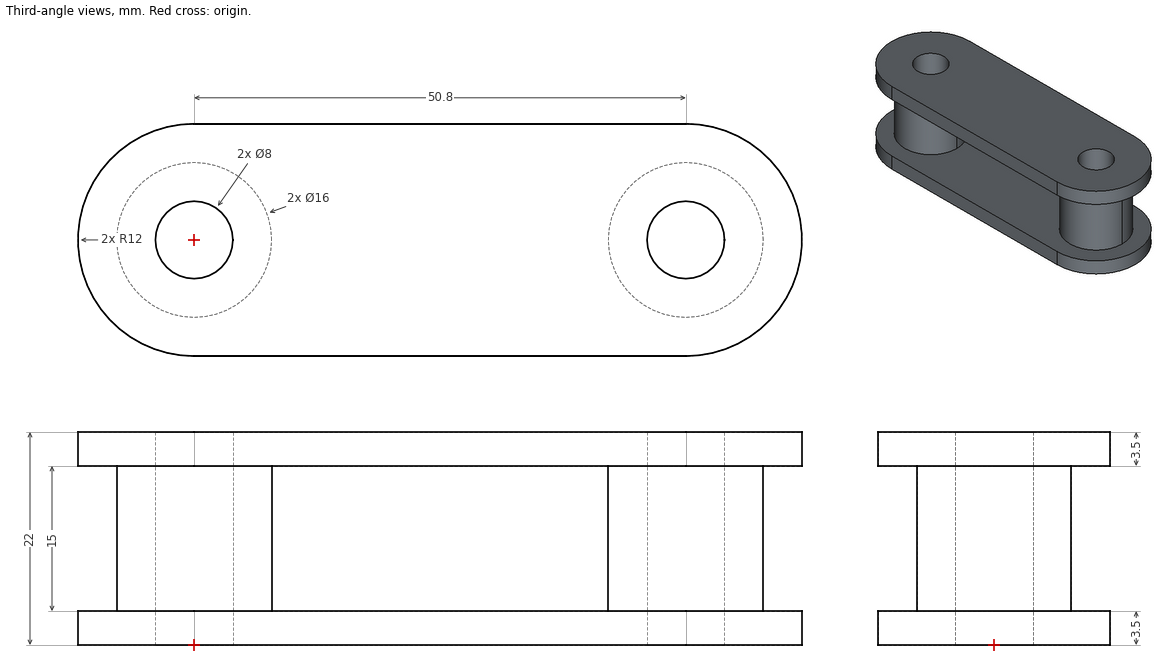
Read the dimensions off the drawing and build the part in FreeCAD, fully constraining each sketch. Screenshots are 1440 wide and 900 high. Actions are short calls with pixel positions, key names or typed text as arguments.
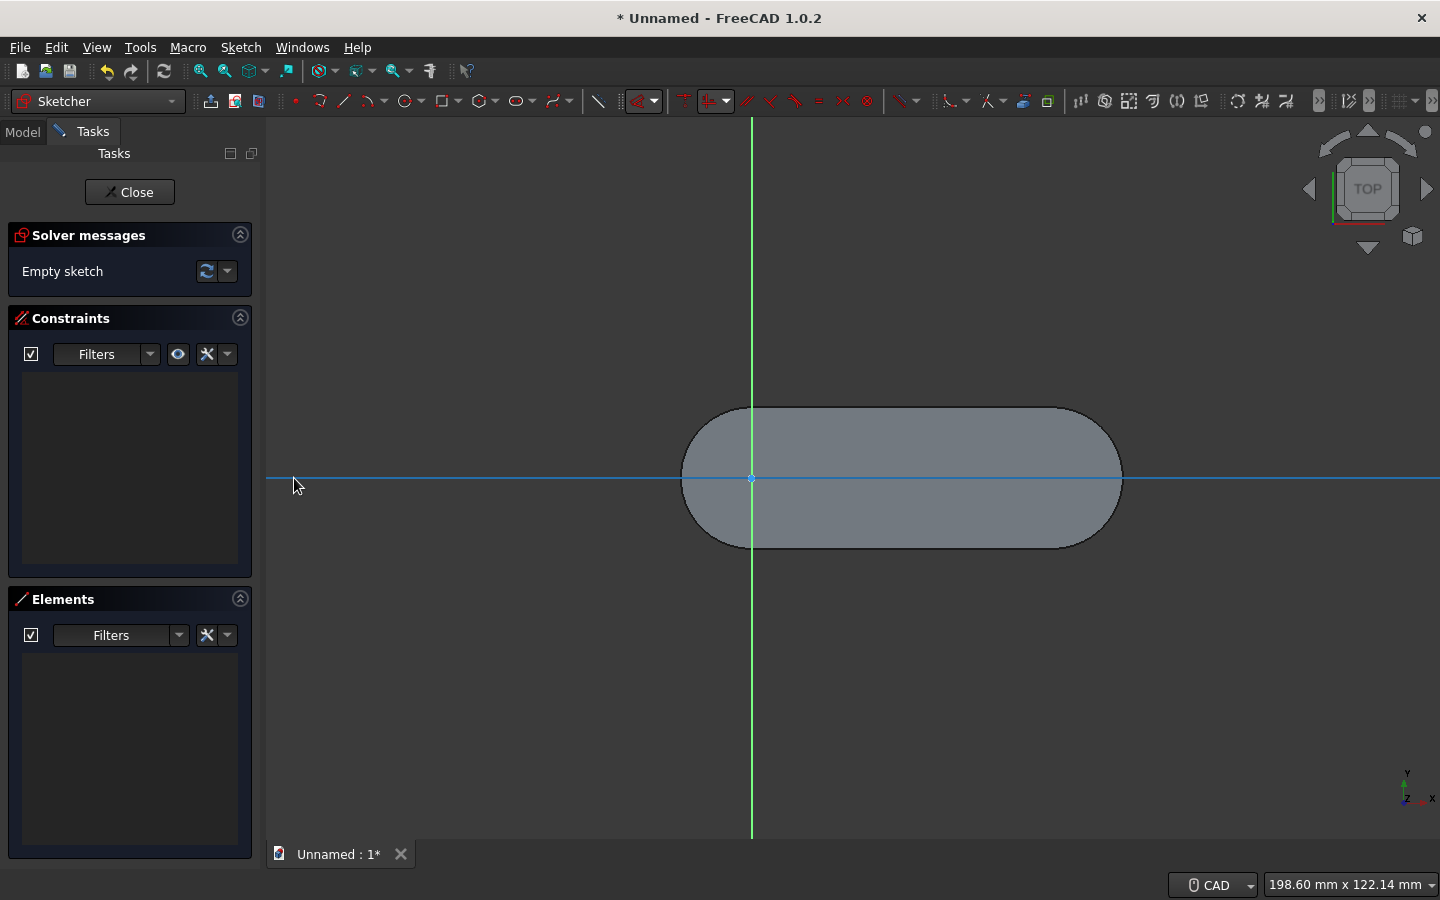
scroll(1045, 478, up, 3)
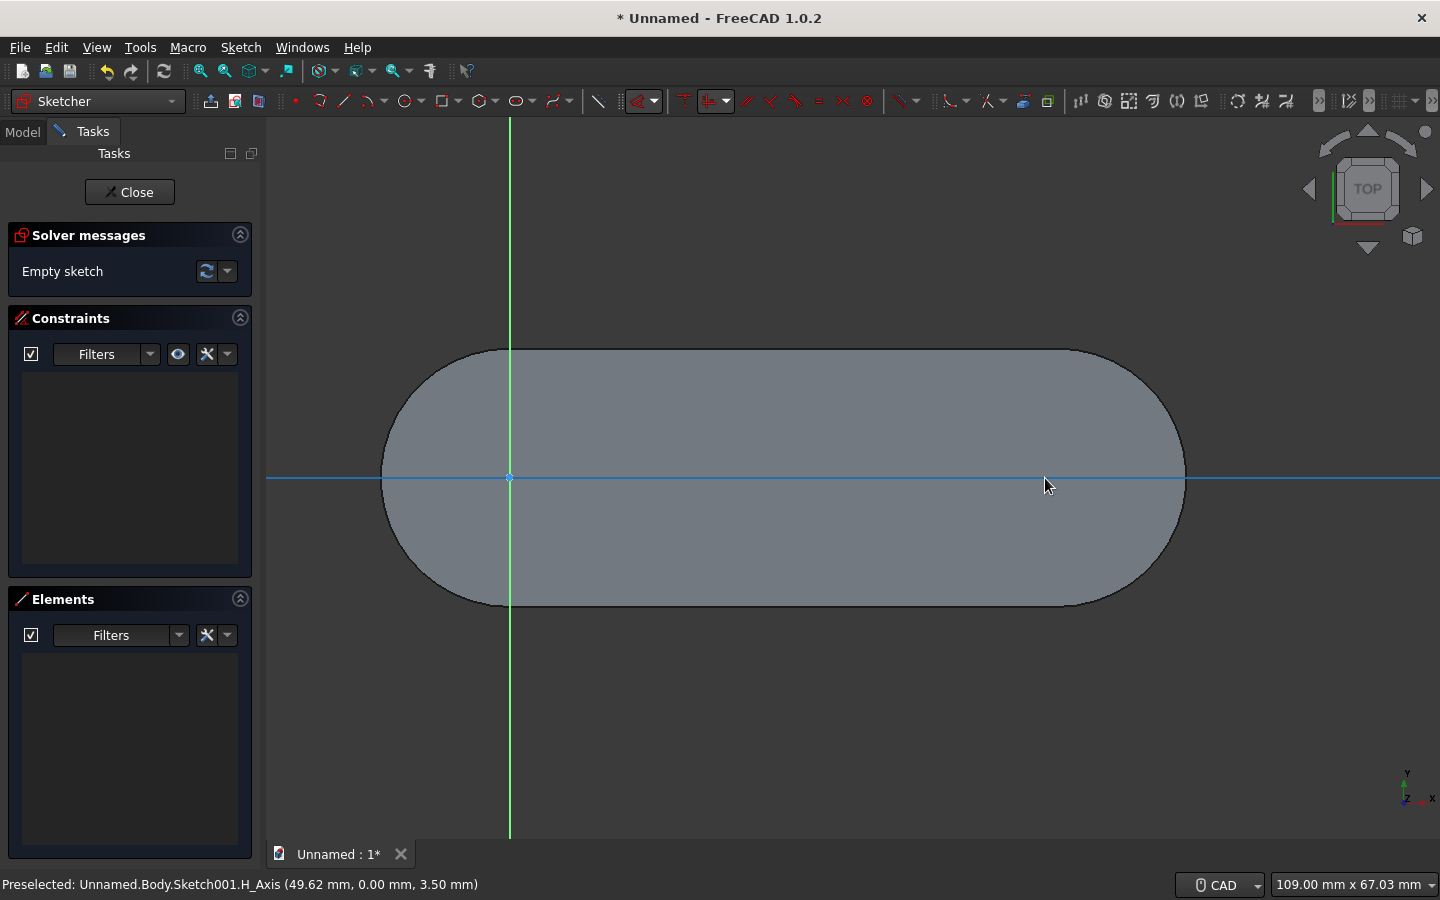
click(406, 102)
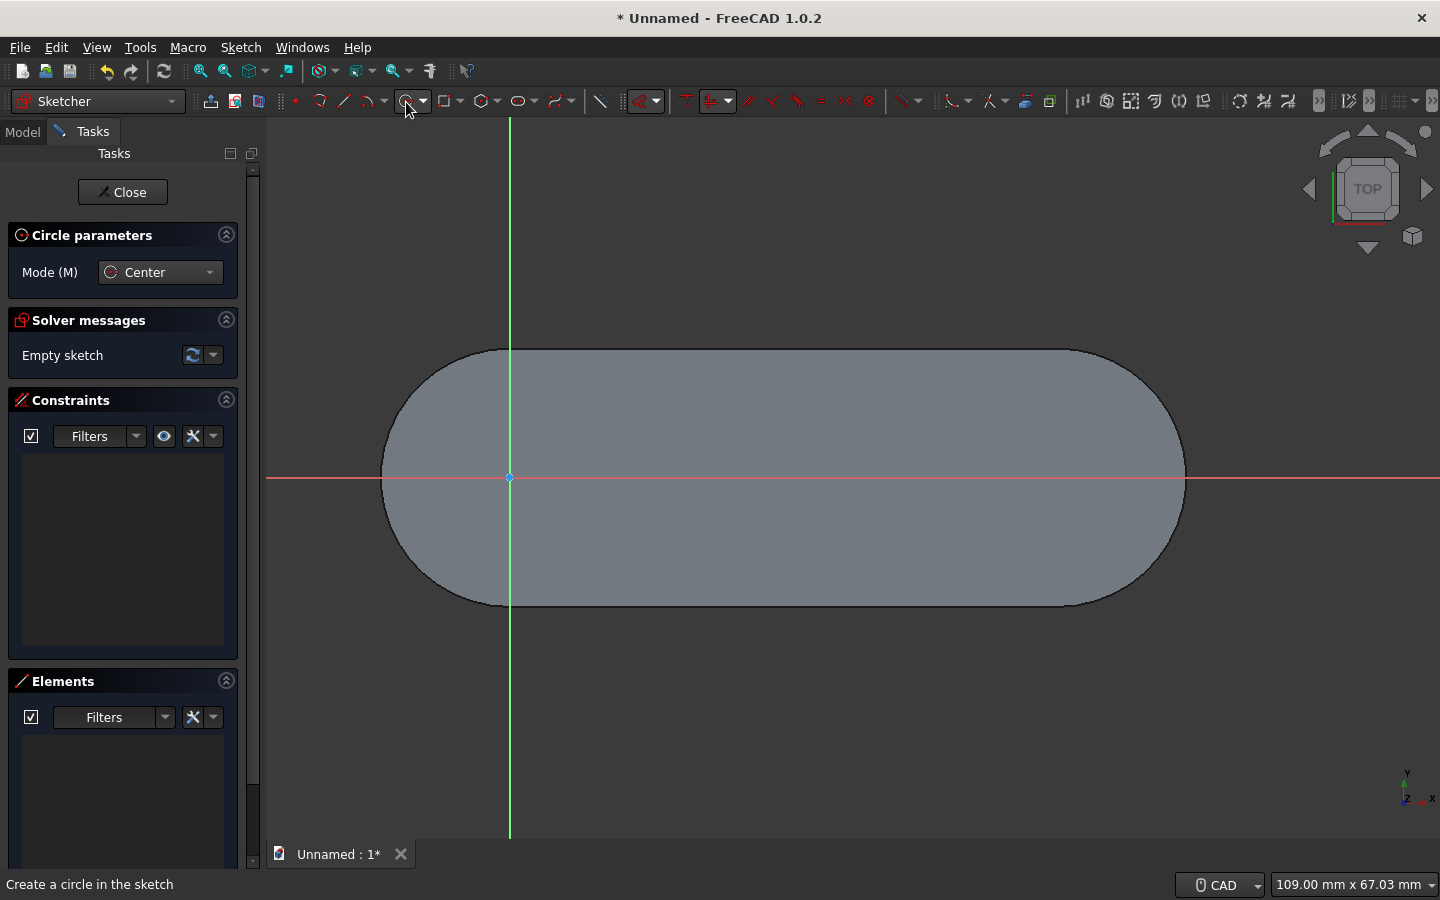
click(510, 478)
move(571, 417)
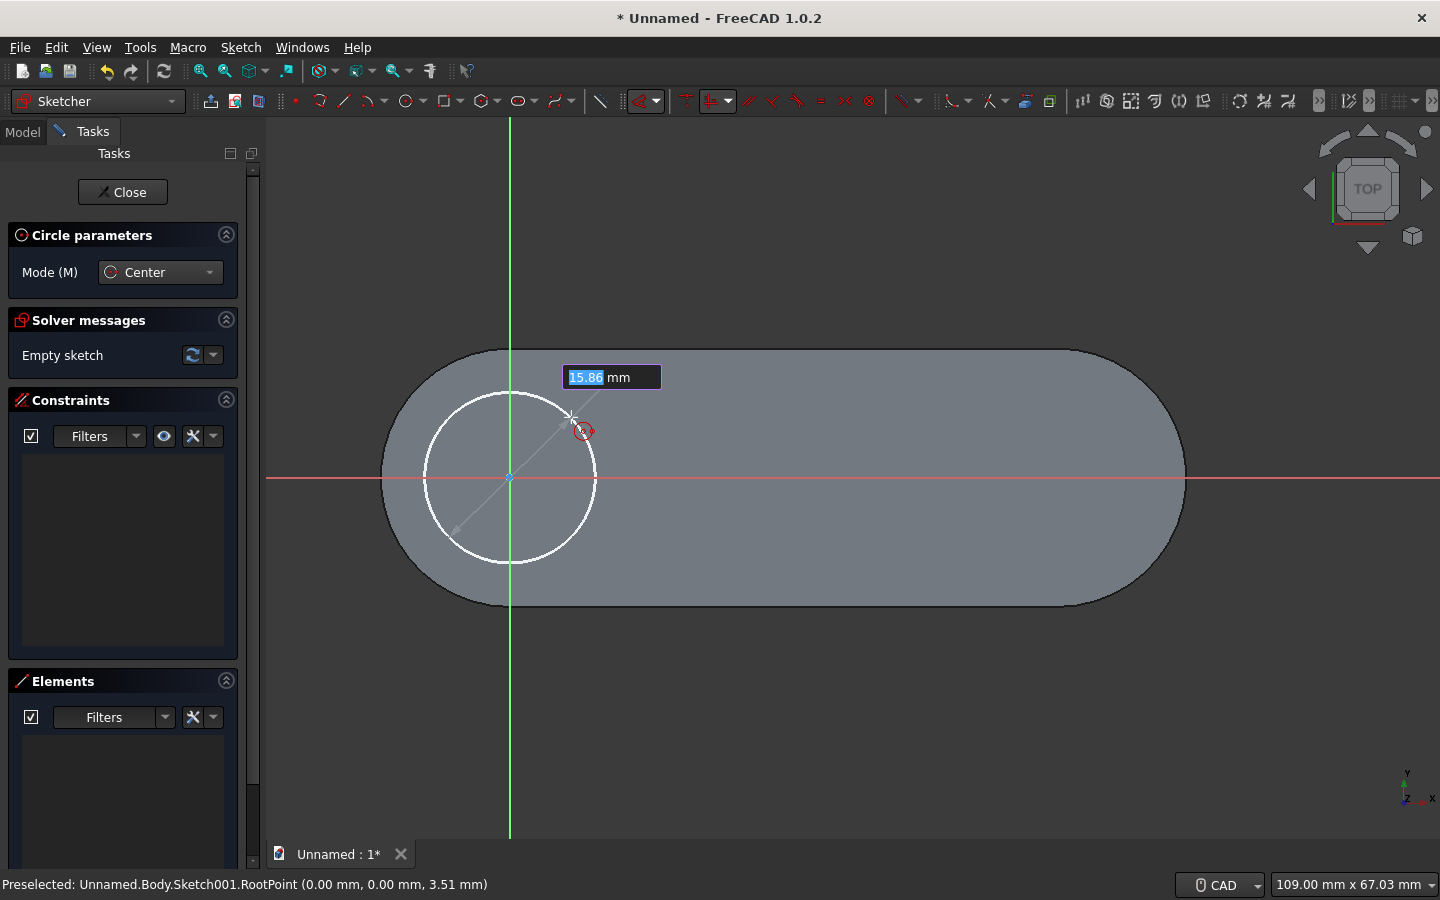
text(16)
key(Return)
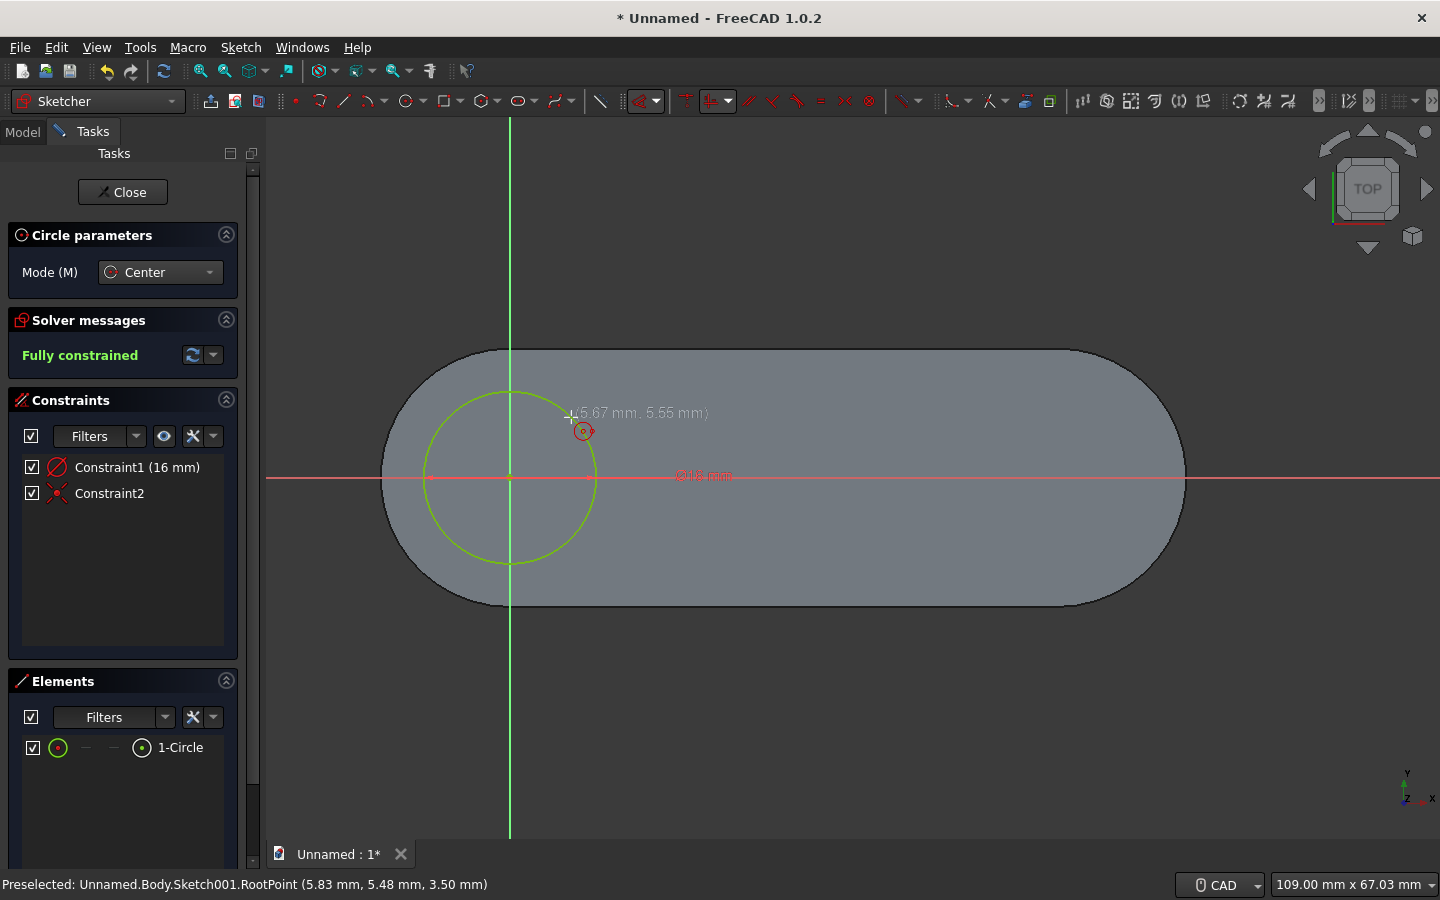
click(1057, 478)
move(1118, 417)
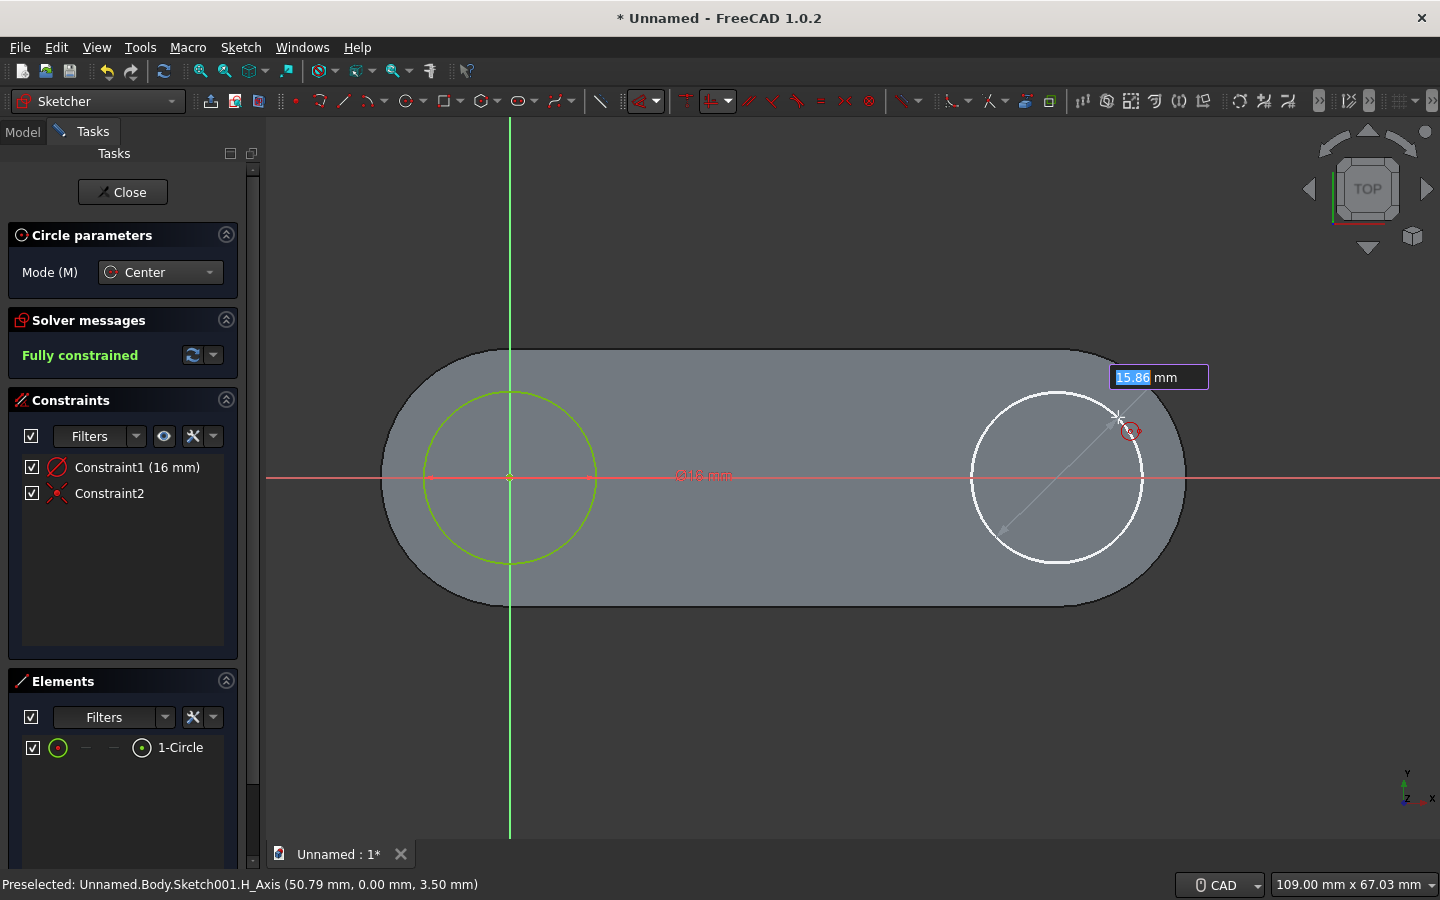
text(16)
key(Return)
key(Escape)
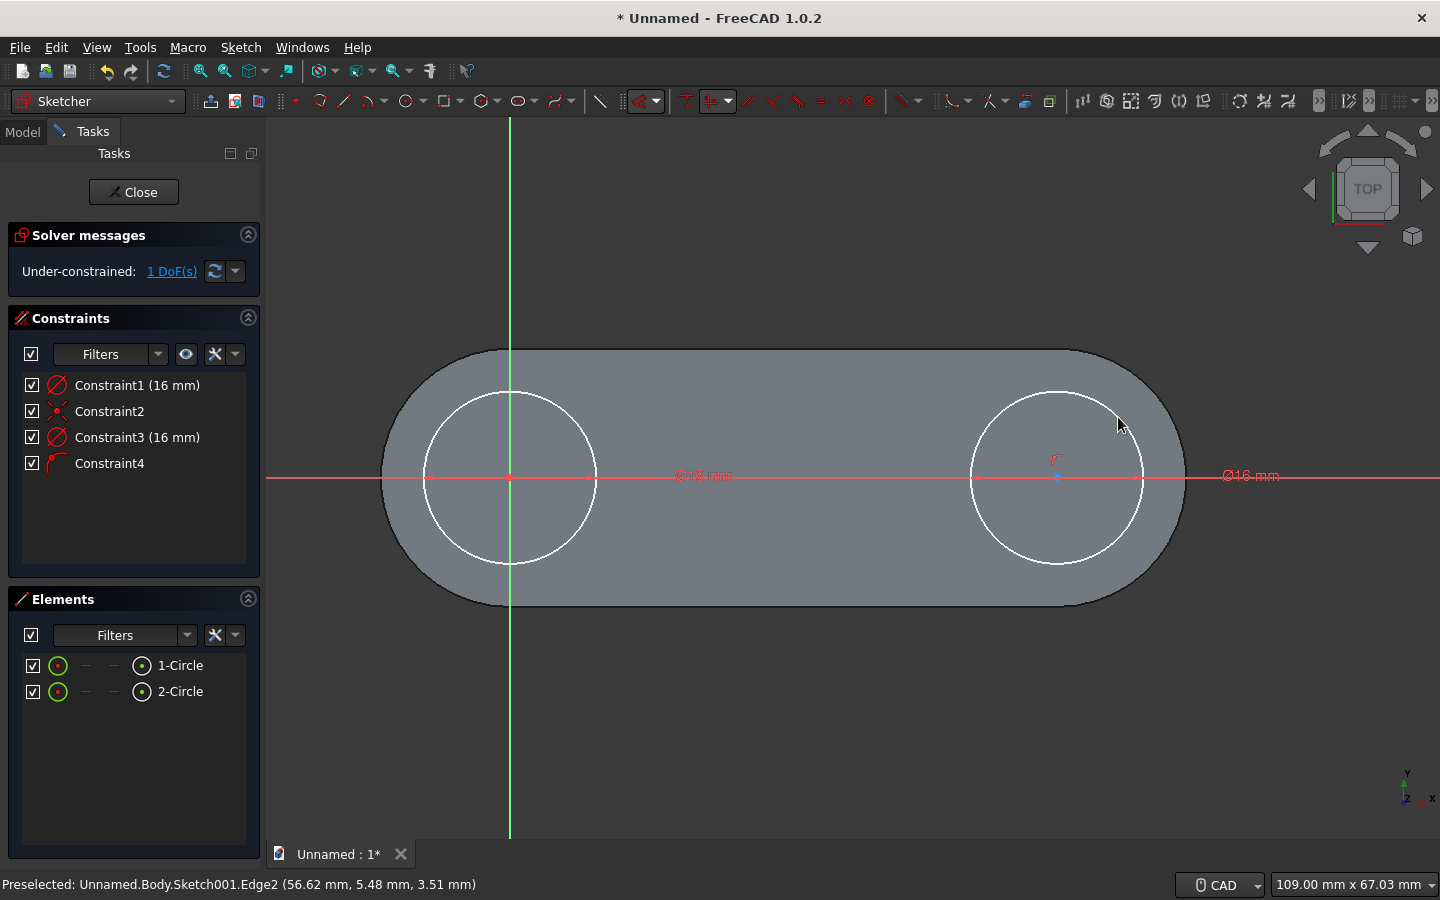
click(1057, 478)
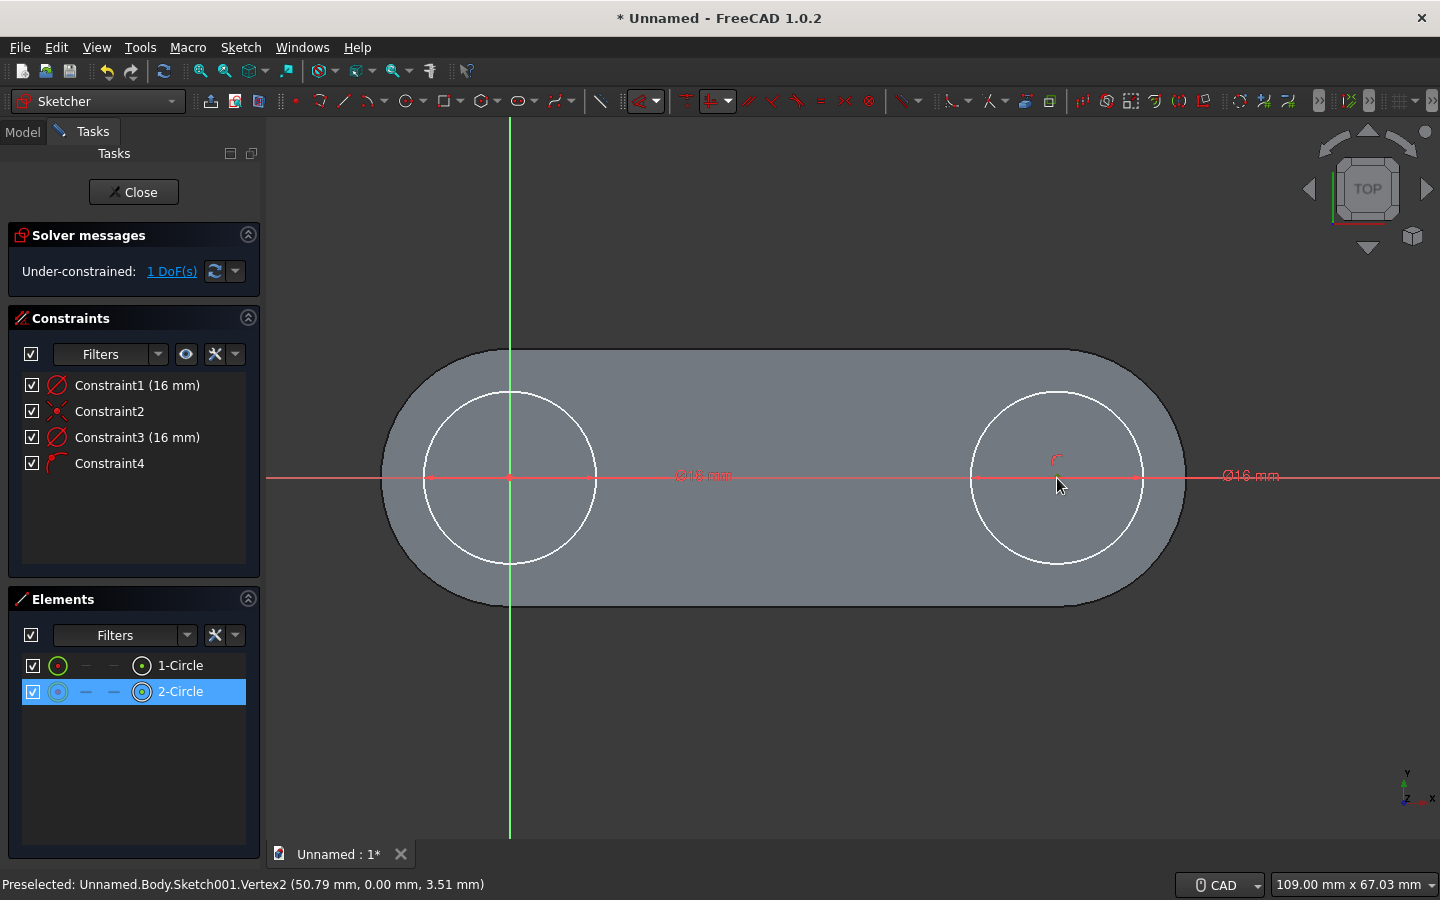
click(658, 102)